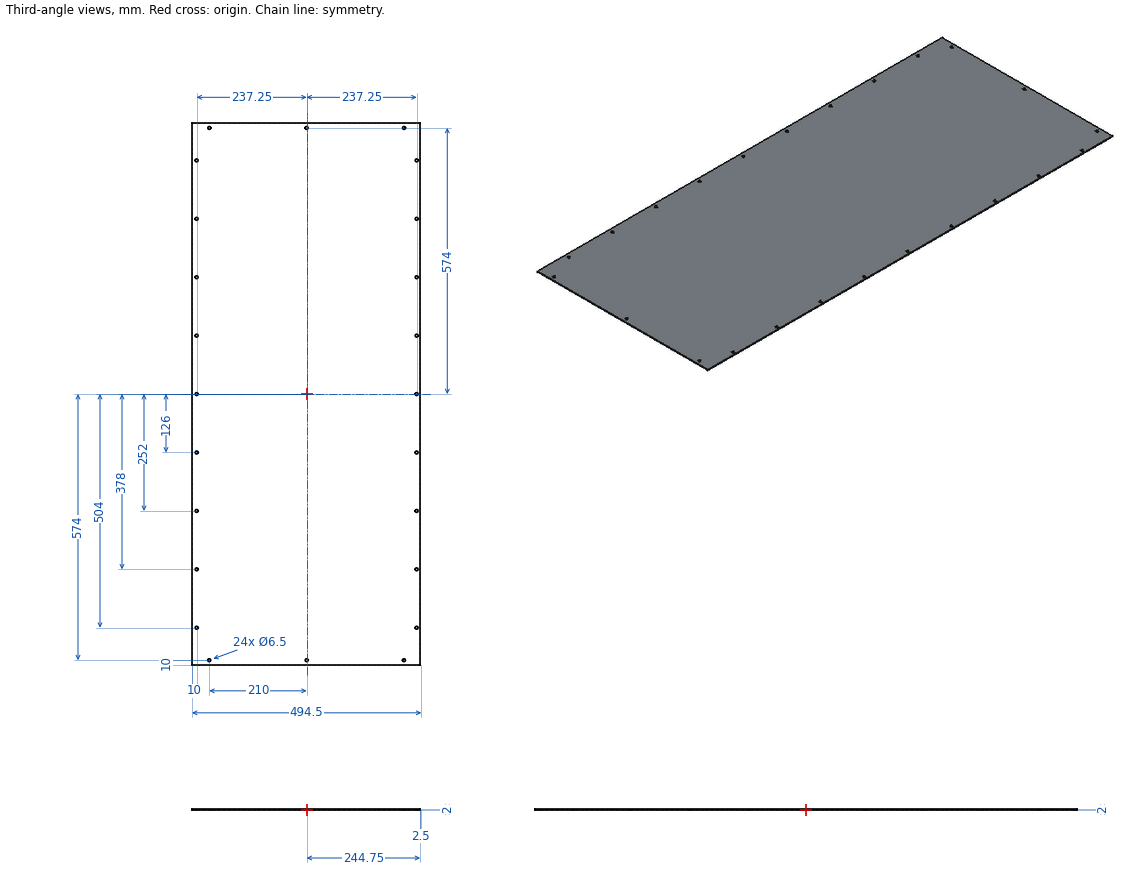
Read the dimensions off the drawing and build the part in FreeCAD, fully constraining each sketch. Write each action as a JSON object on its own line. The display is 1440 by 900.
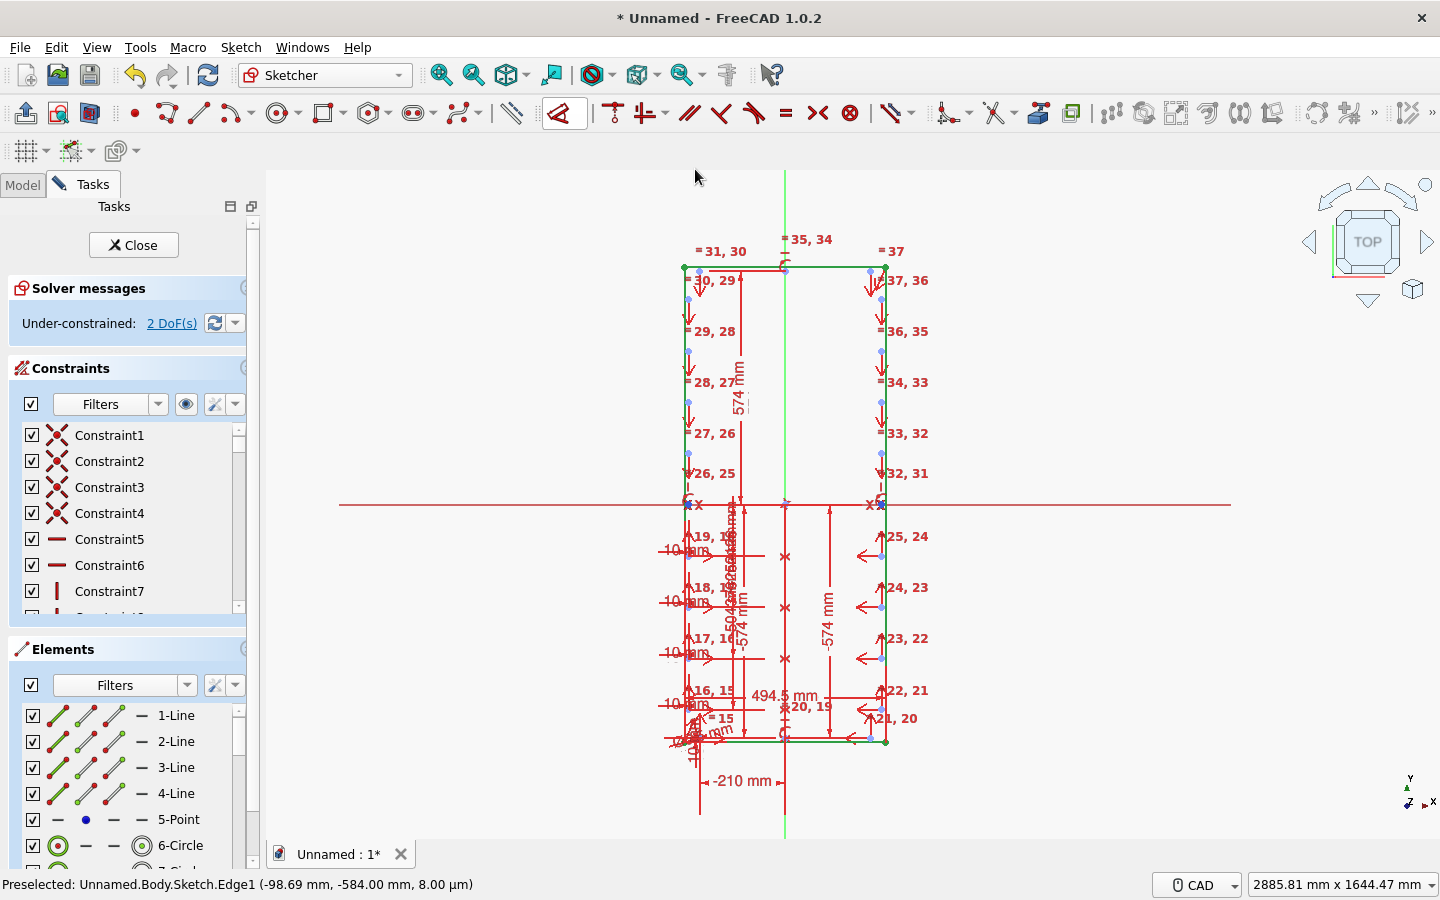
{"action": "left_click", "coordinate": [689, 505]}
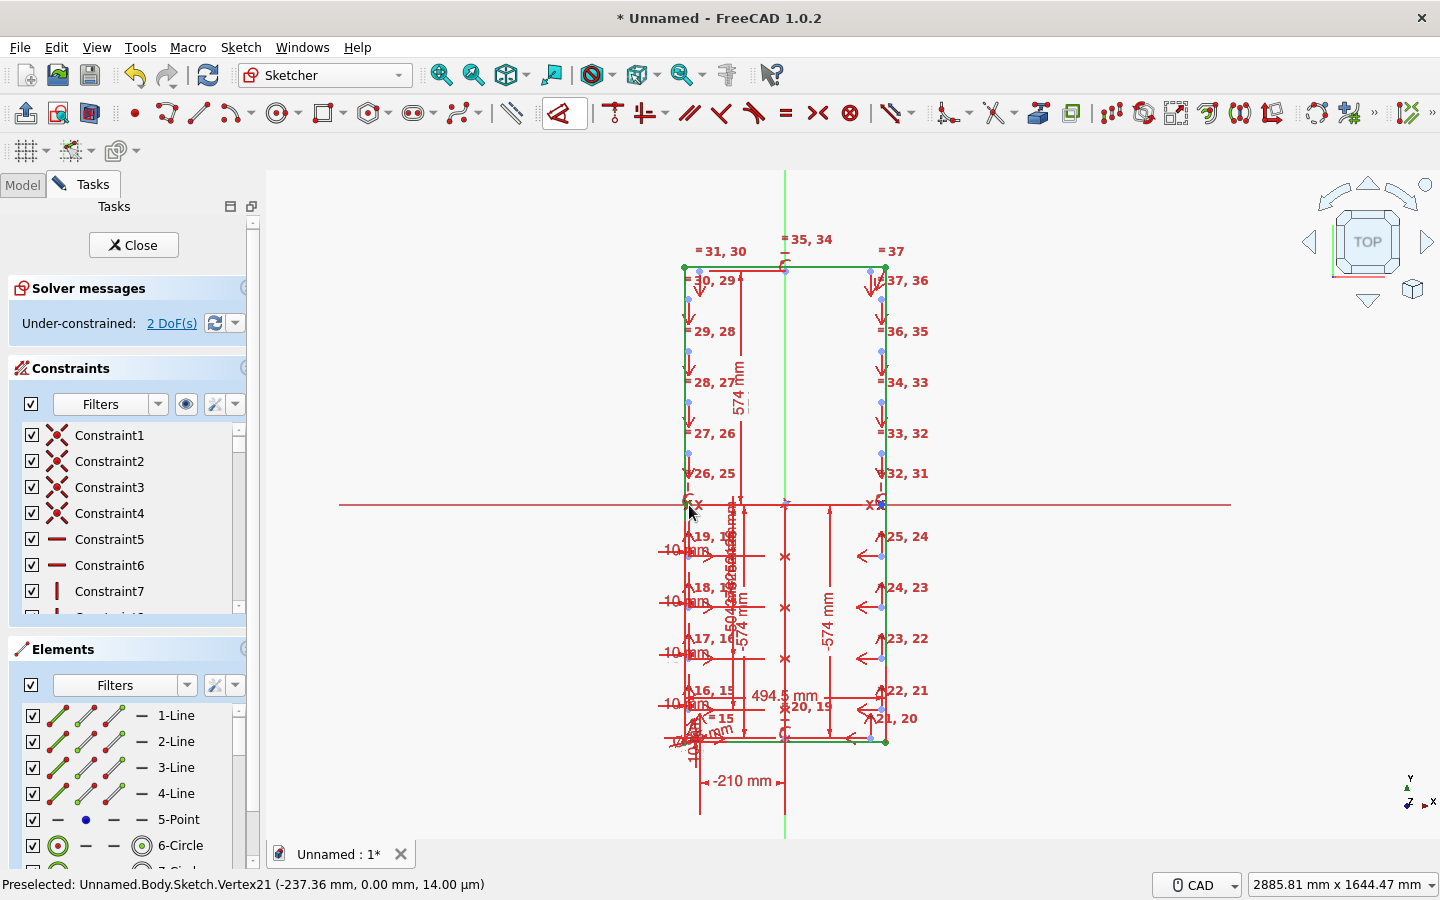
{"action": "key", "text": "l"}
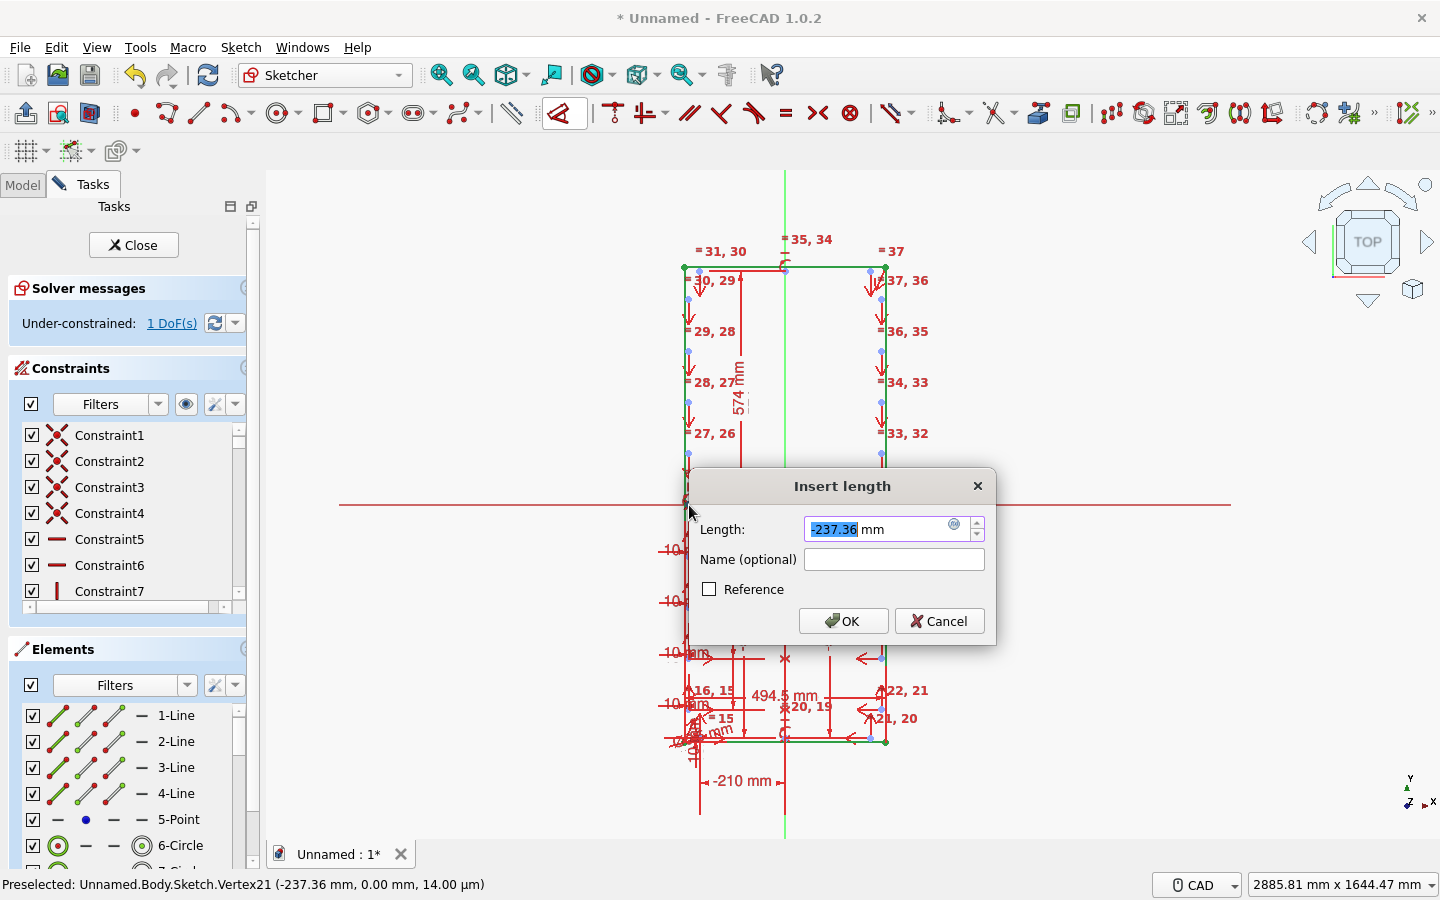
{"action": "type", "text": "-237.25"}
{"action": "key", "text": "Return"}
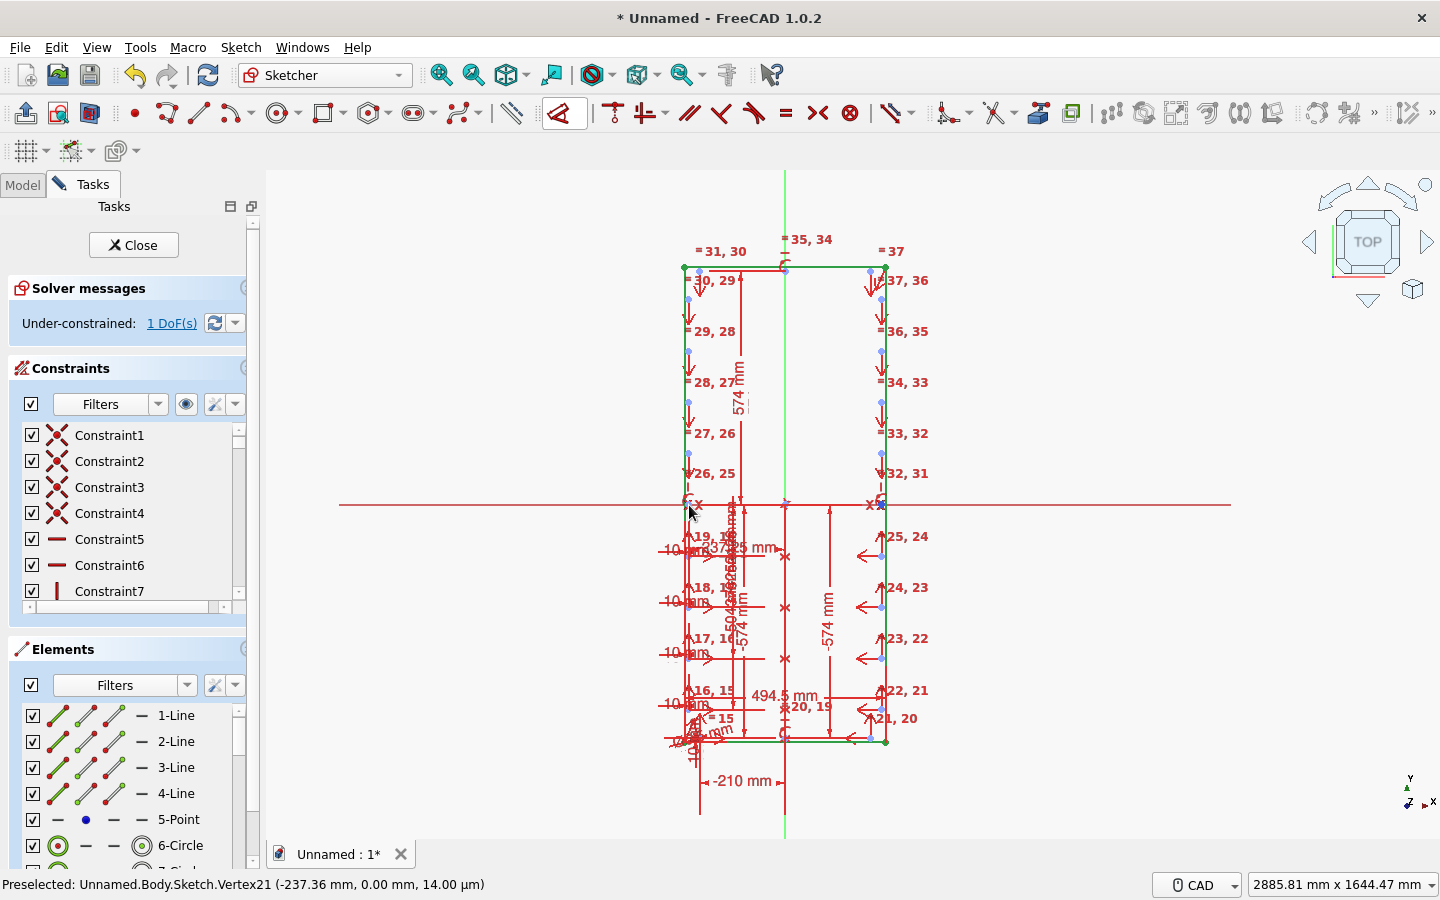
{"action": "left_click", "coordinate": [882, 505]}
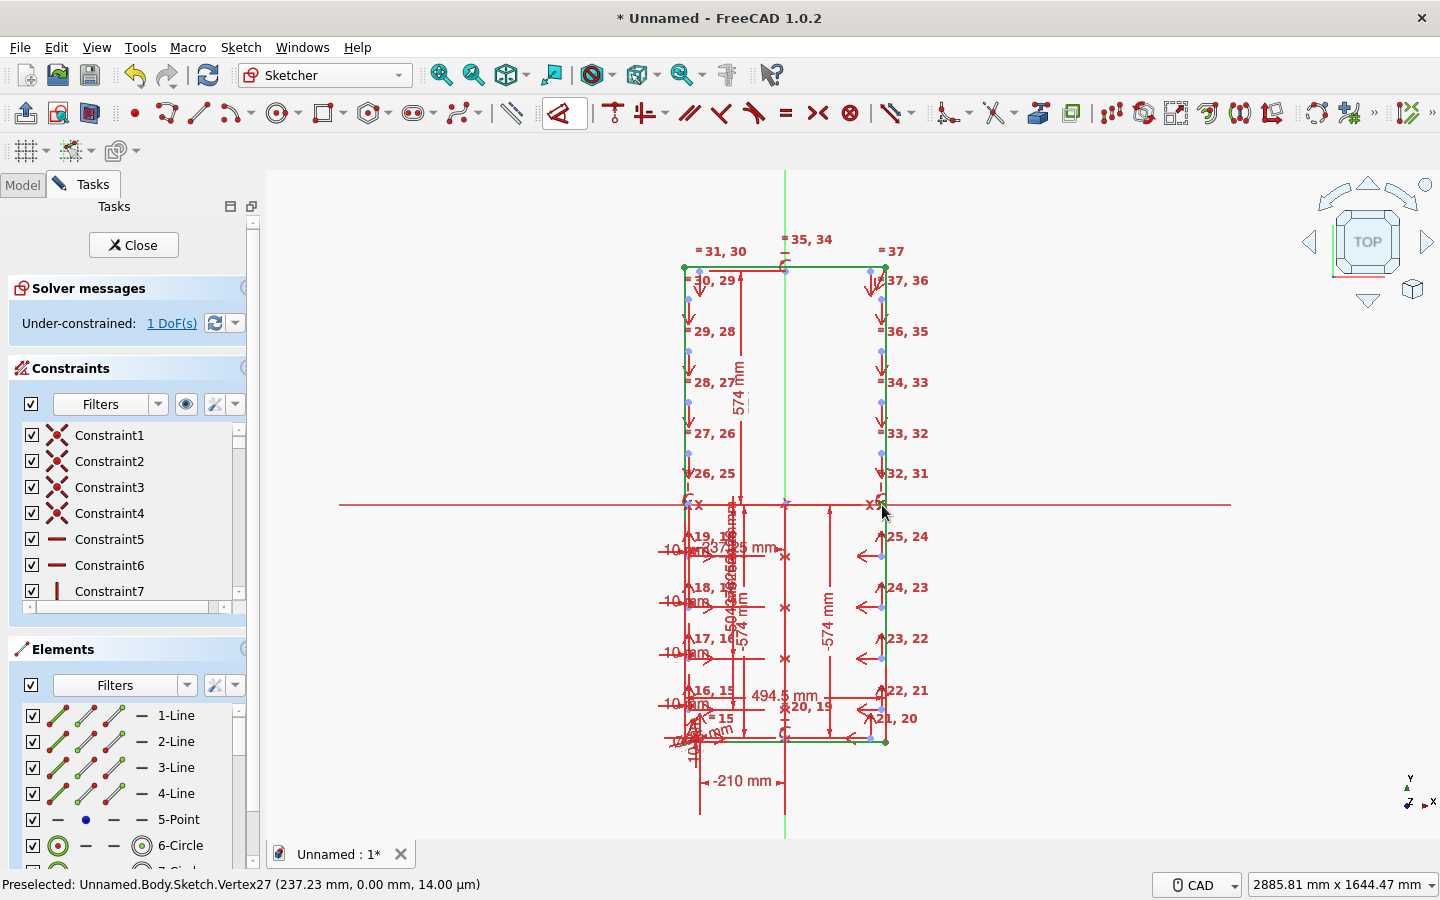
{"action": "key", "text": "l"}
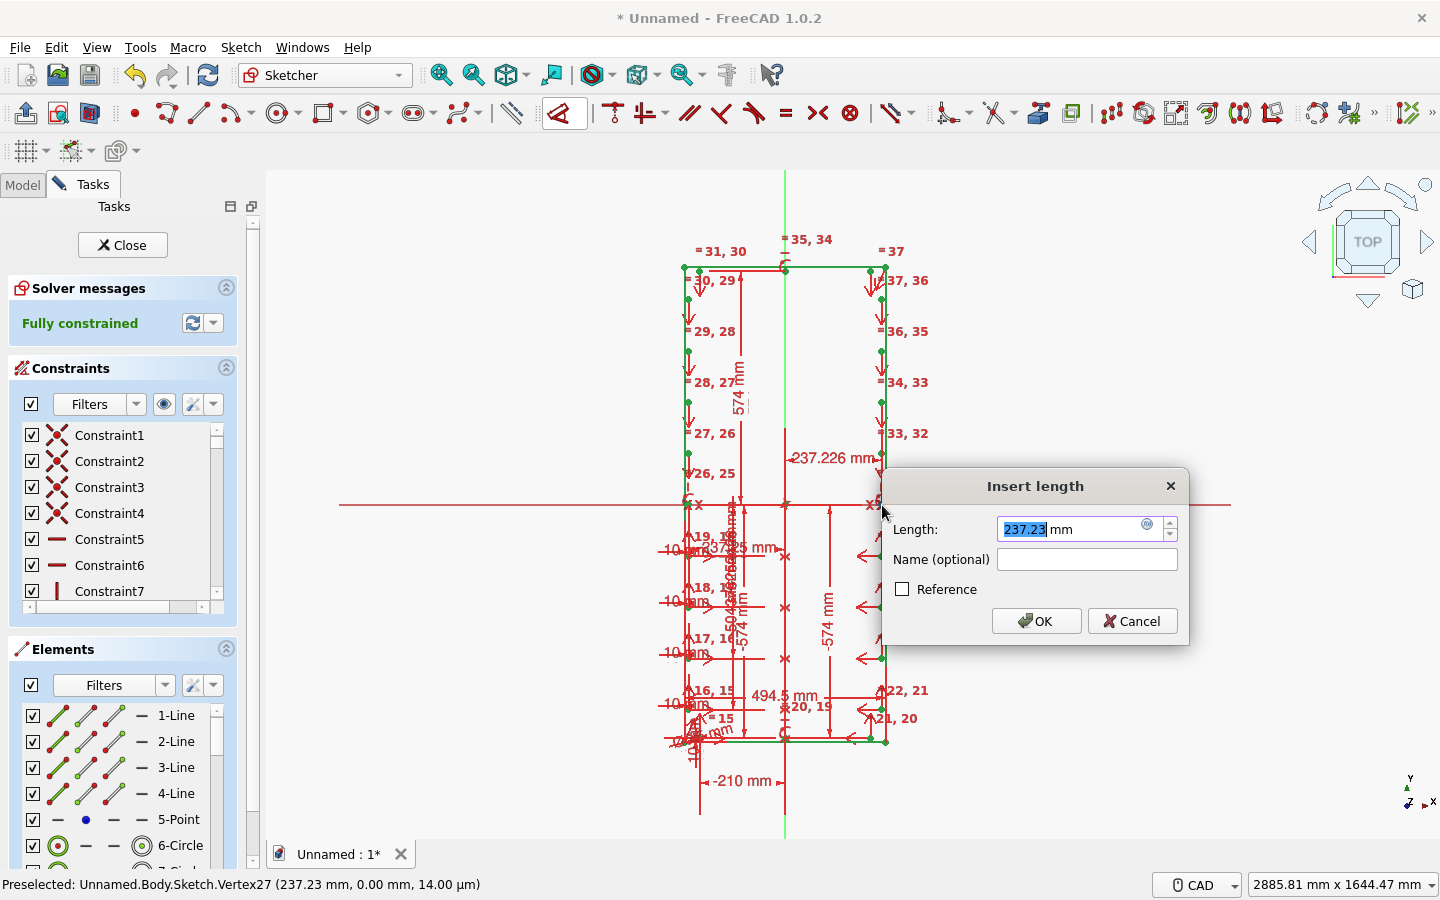
{"action": "type", "text": "237.25"}
{"action": "key", "text": "Return"}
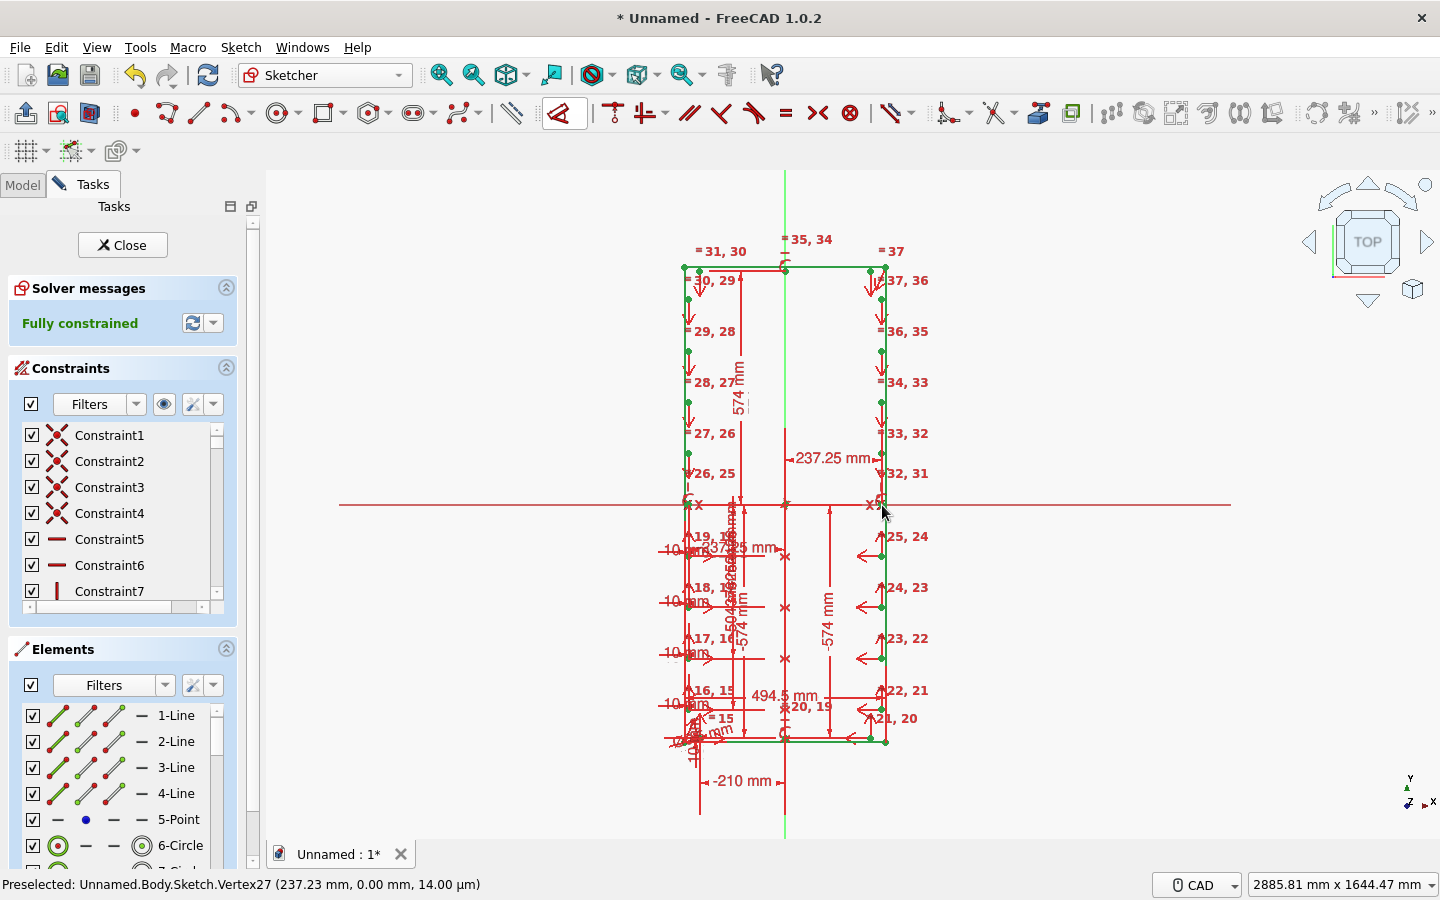
{"action": "left_click", "coordinate": [123, 245]}